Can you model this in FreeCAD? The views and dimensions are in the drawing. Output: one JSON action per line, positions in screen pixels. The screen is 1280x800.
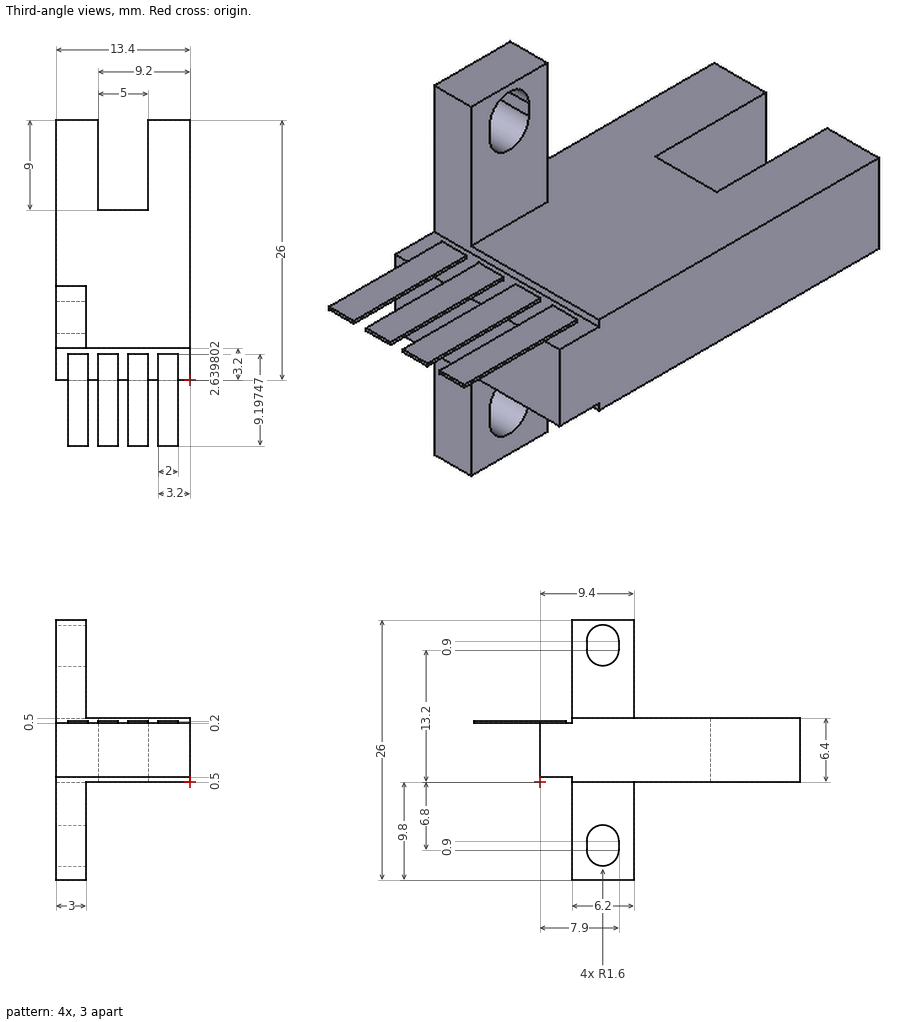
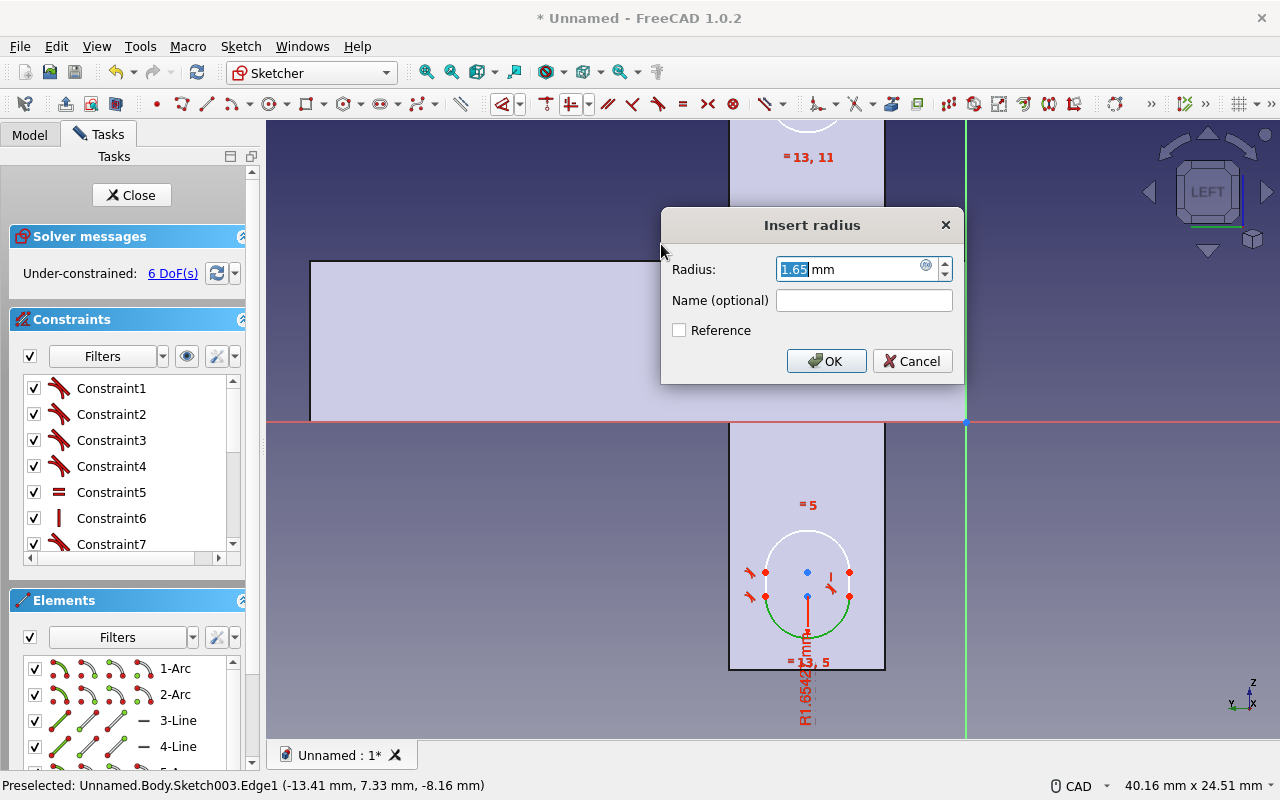
{"action": "type", "text": "1.6"}
{"action": "key", "text": "Return"}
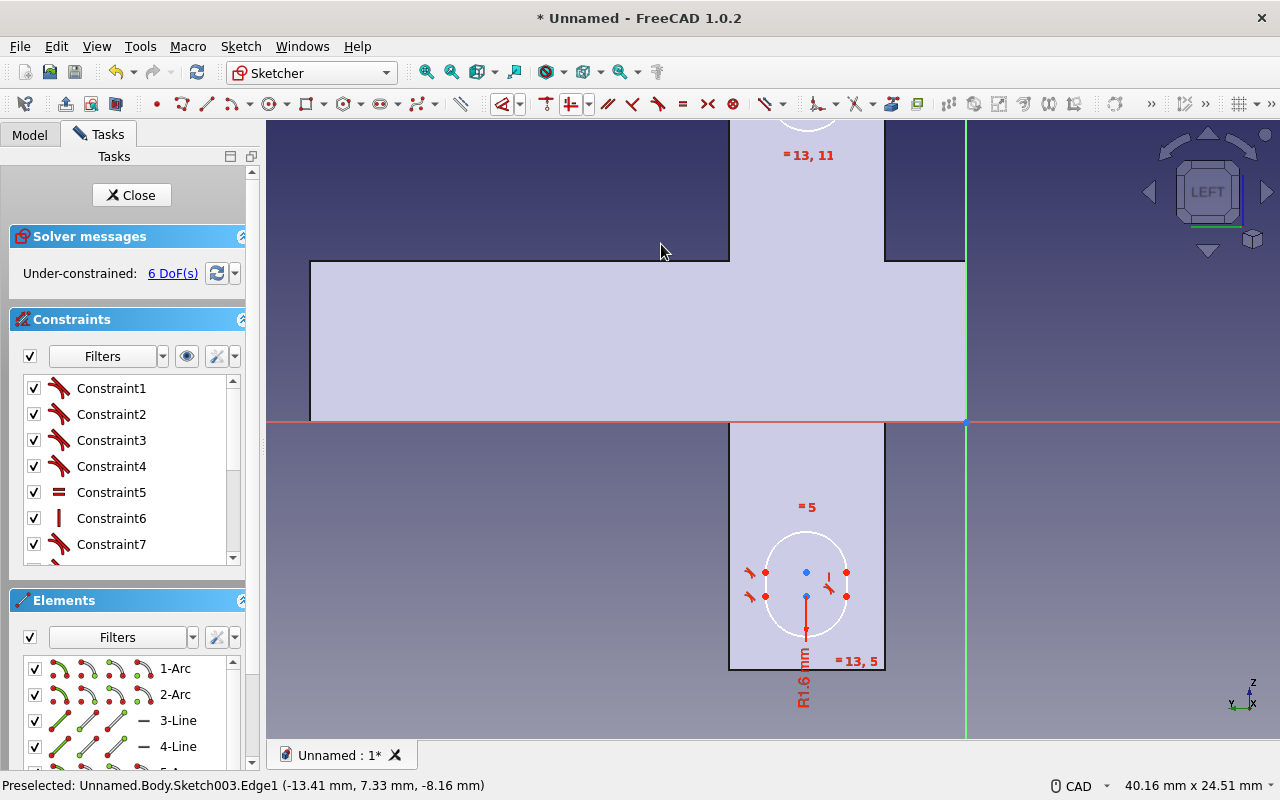
{"action": "scroll", "coordinate": [766, 587], "scroll_direction": "up", "scroll_amount": 3}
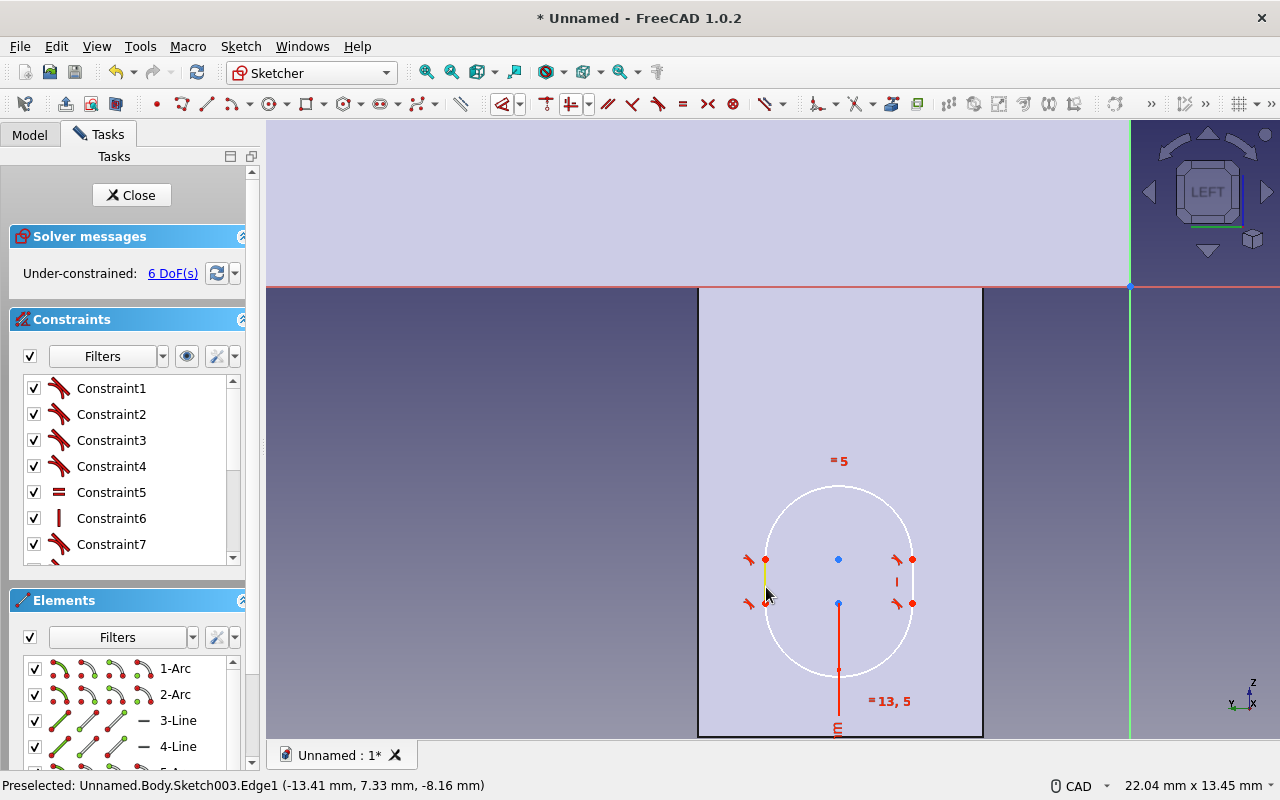
{"action": "left_click", "coordinate": [765, 586]}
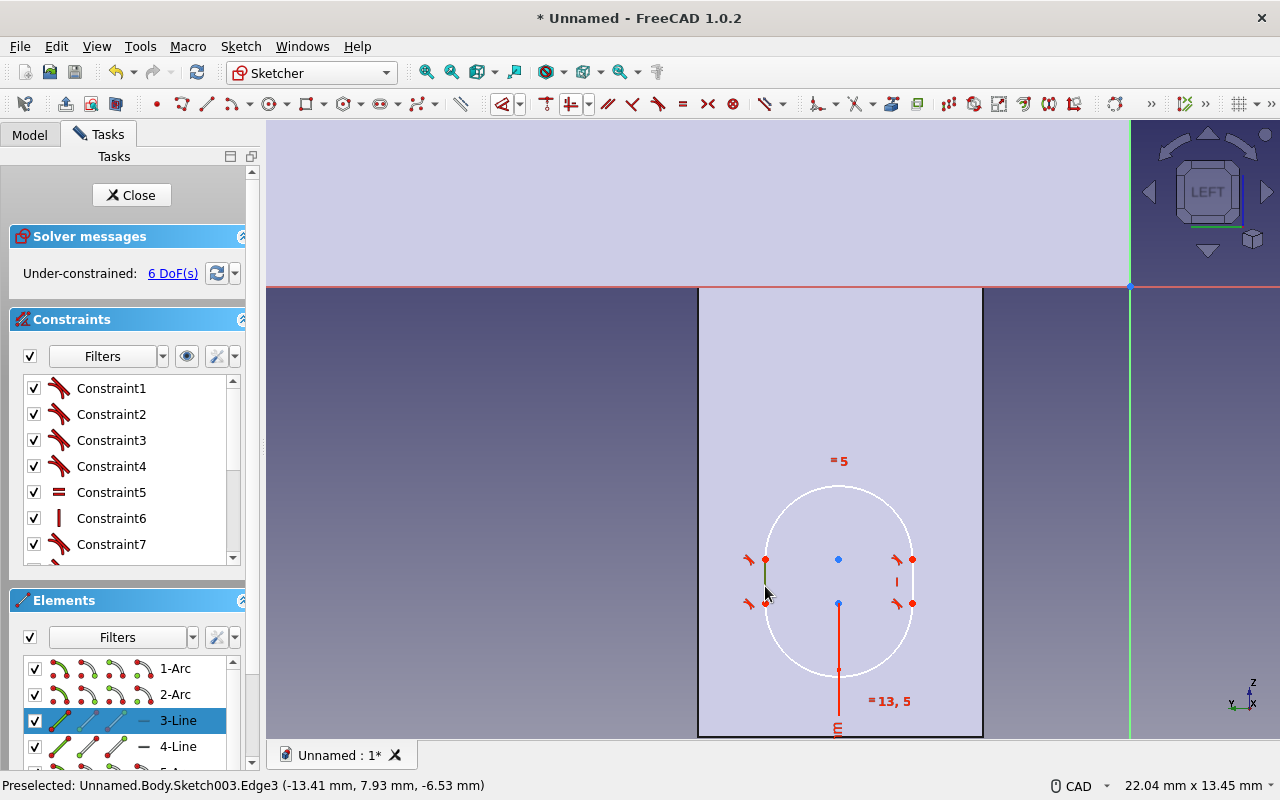
{"action": "key", "text": "i"}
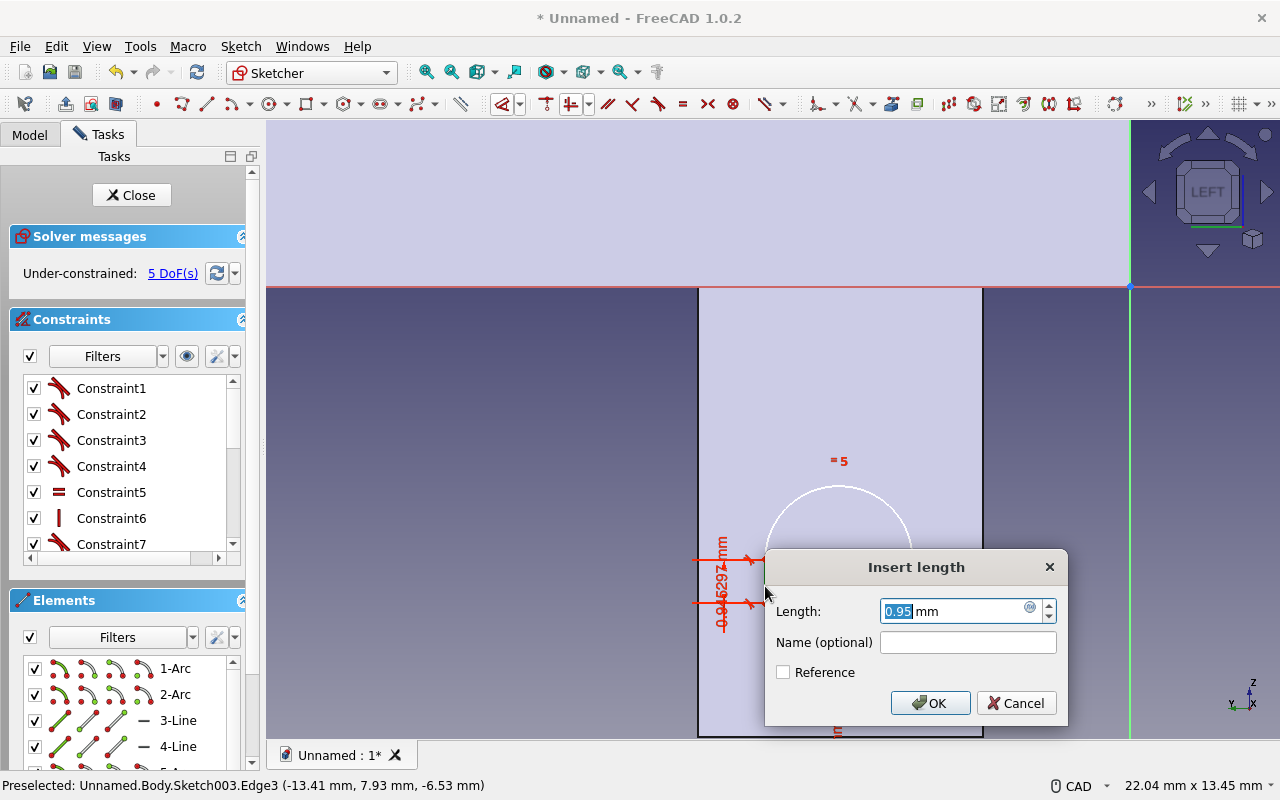
{"action": "type", "text": "0.9"}
{"action": "key", "text": "Return"}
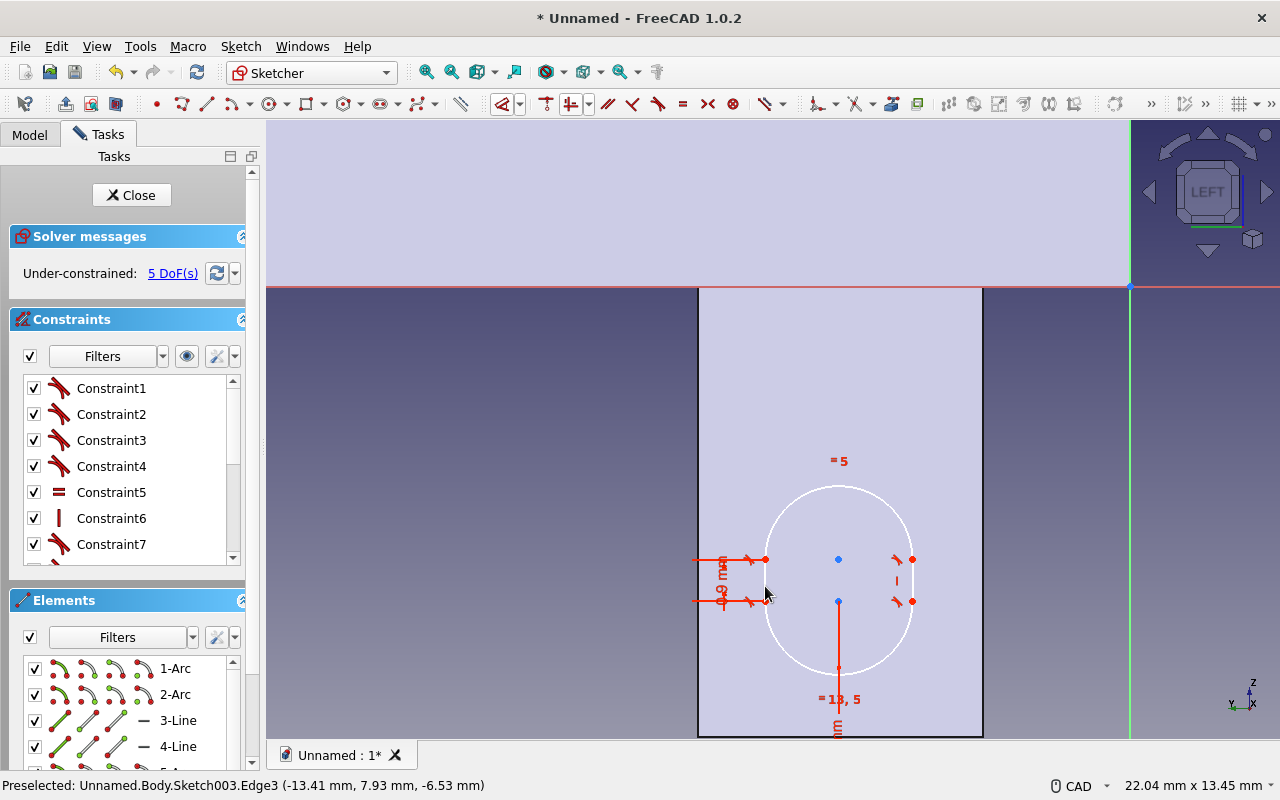
{"action": "scroll", "coordinate": [563, 610], "scroll_direction": "down", "scroll_amount": 5}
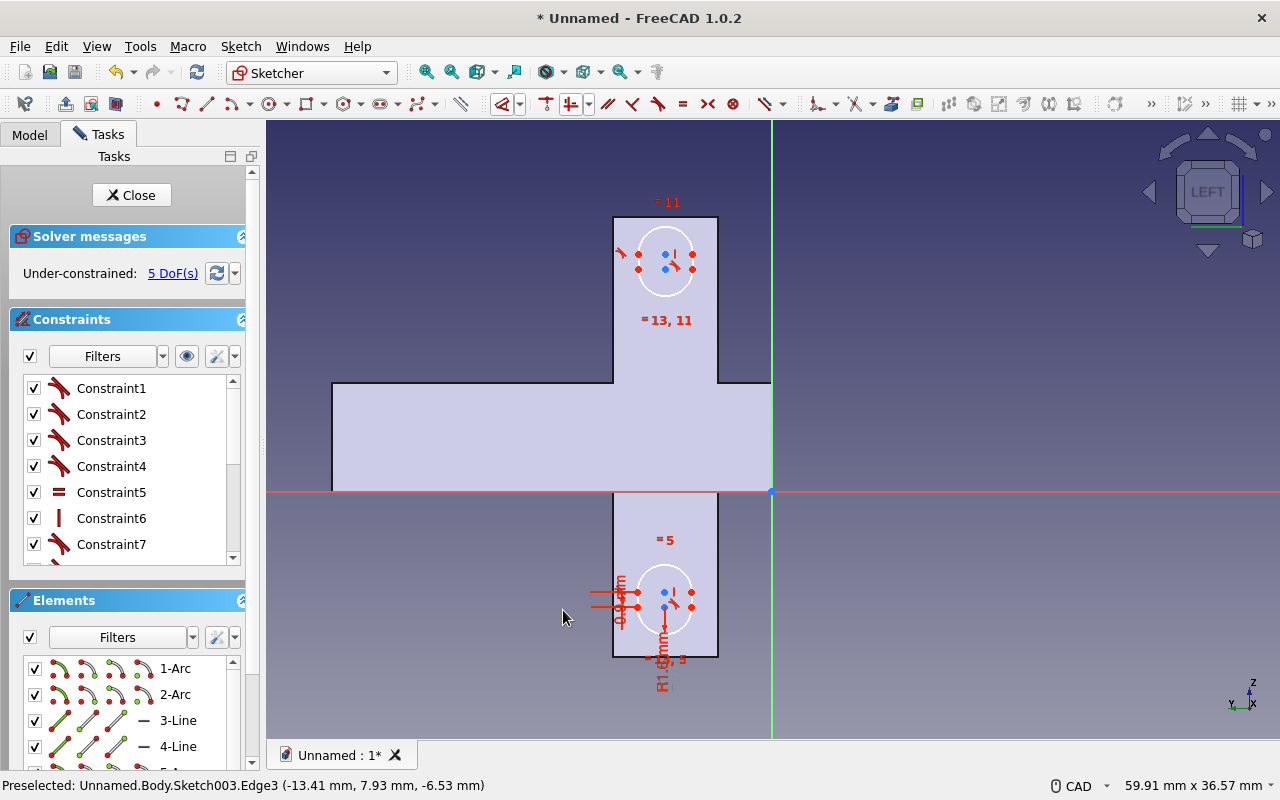
{"action": "scroll", "coordinate": [639, 265], "scroll_direction": "up", "scroll_amount": 6}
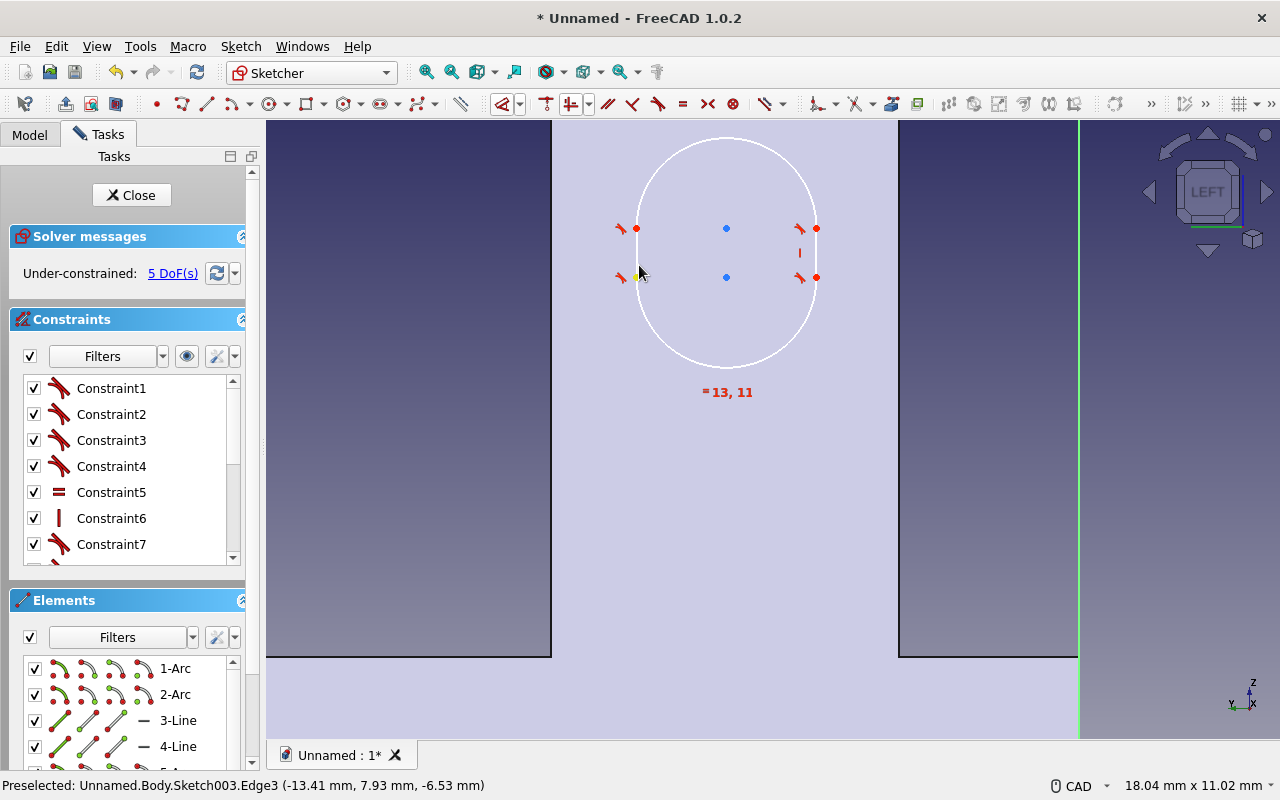
{"action": "left_click", "coordinate": [637, 263]}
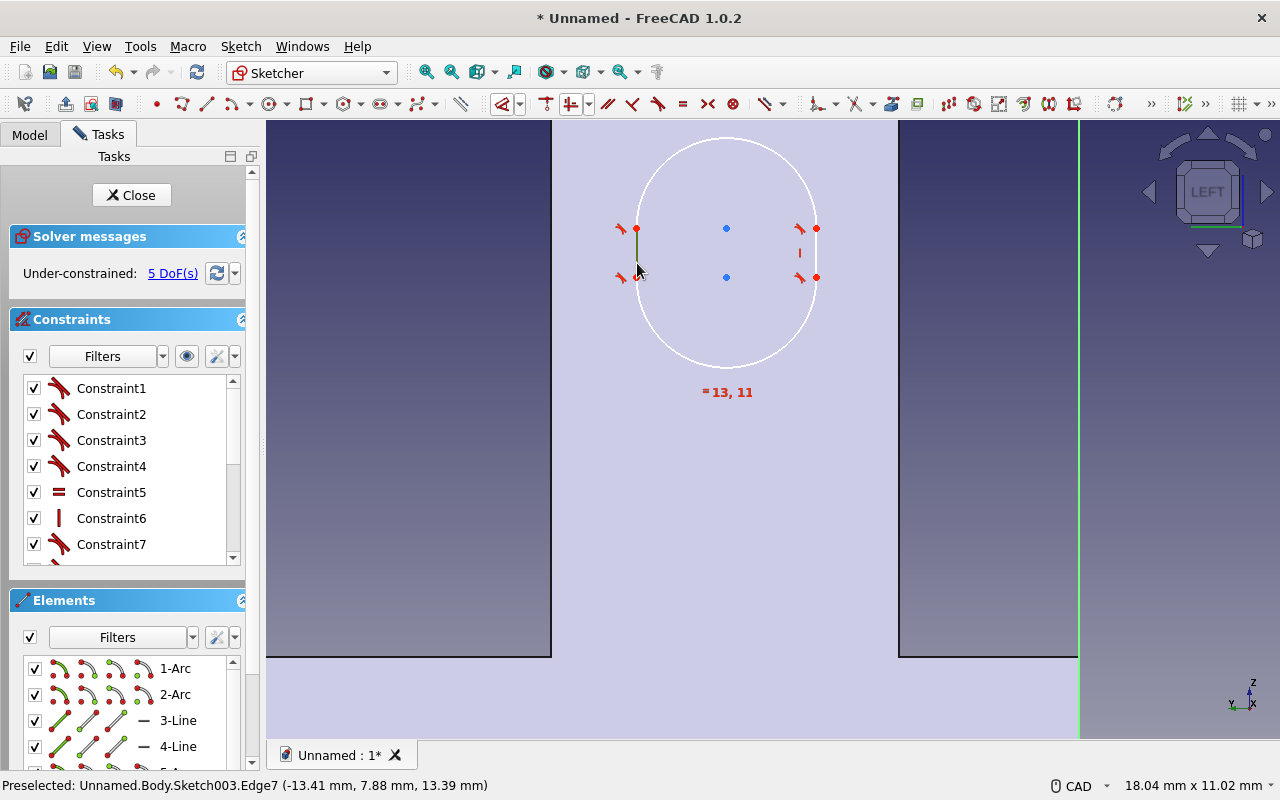
{"action": "left_click", "coordinate": [520, 104]}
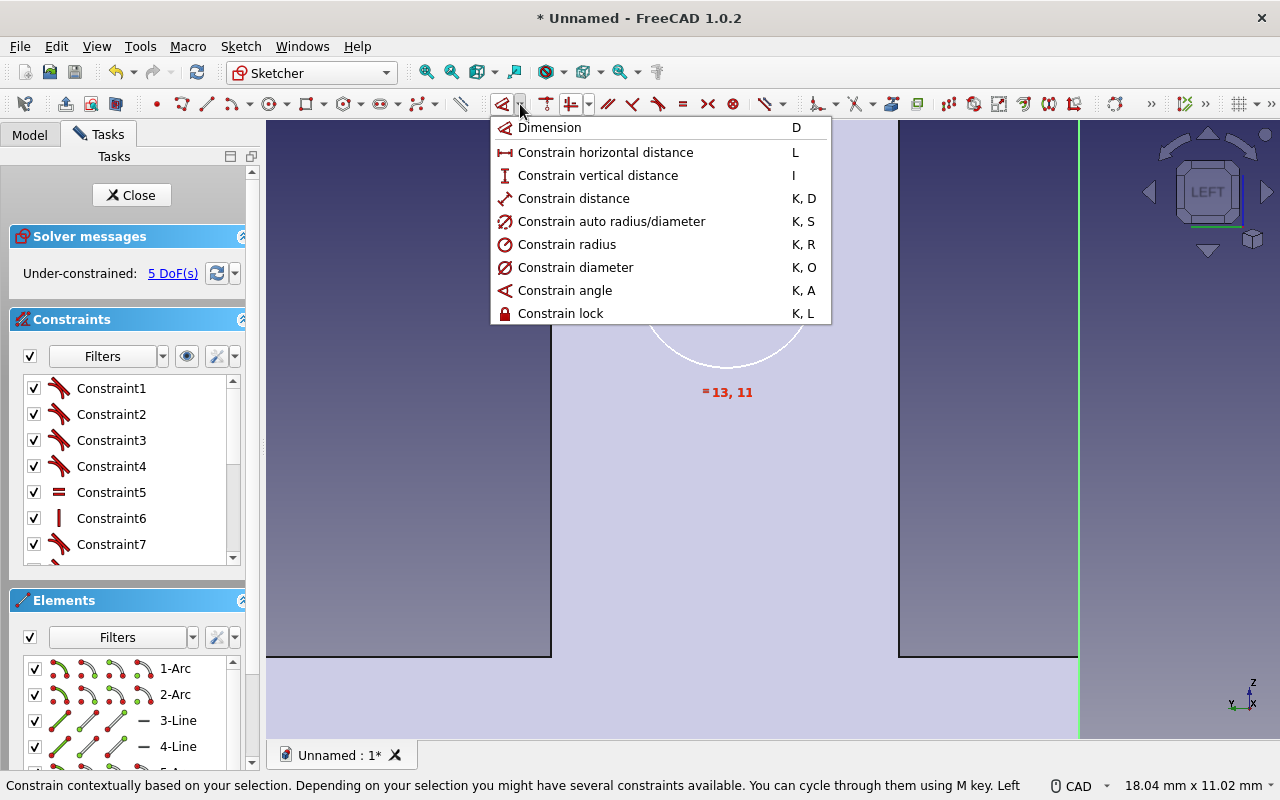
{"action": "left_click", "coordinate": [661, 176]}